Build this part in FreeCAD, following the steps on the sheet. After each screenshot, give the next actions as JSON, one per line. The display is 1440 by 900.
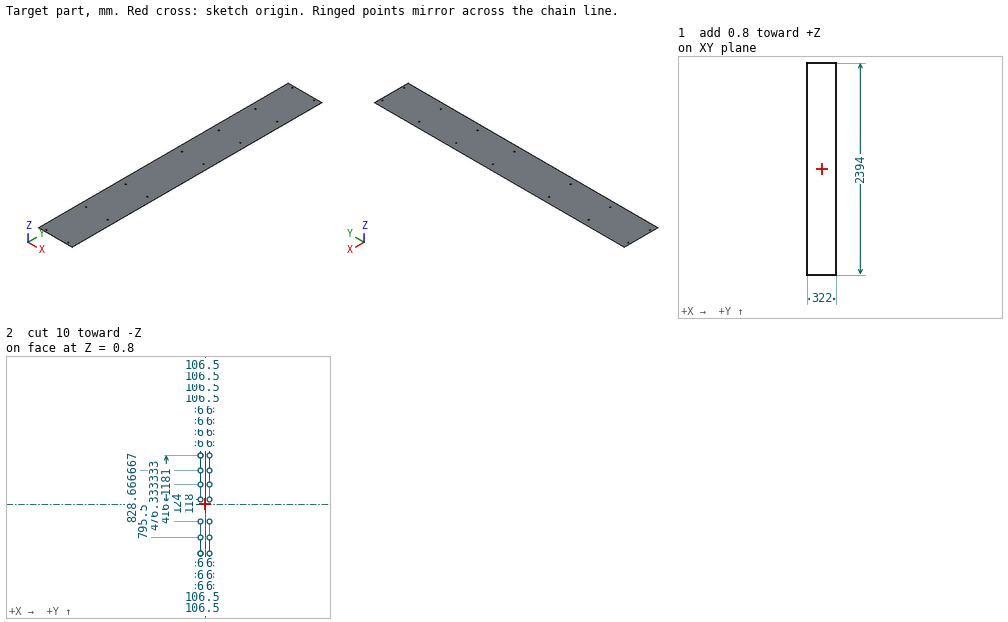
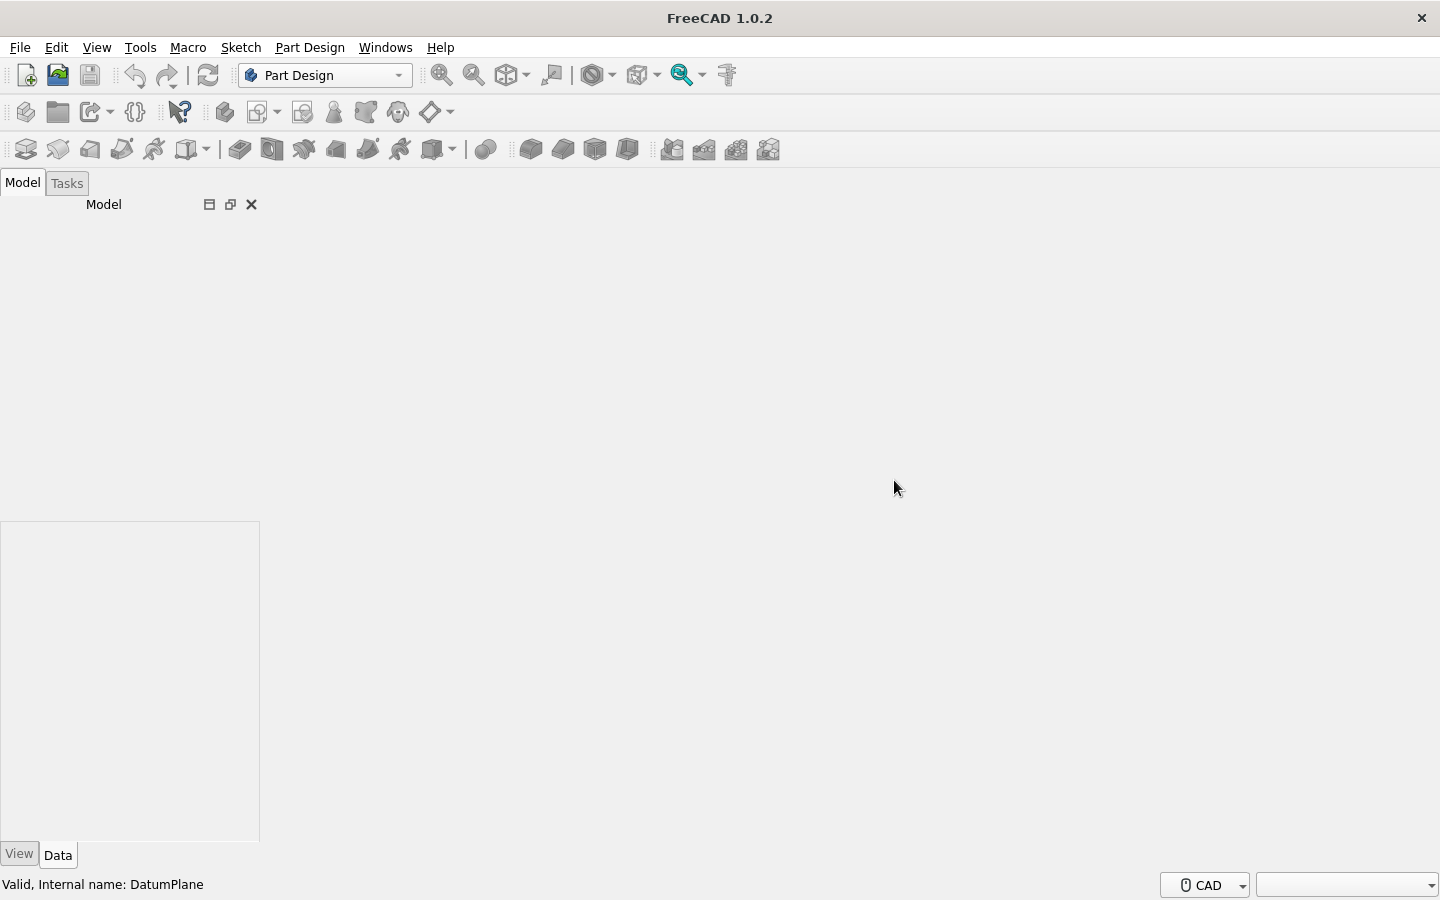
{"action": "left_click", "coordinate": [26, 76]}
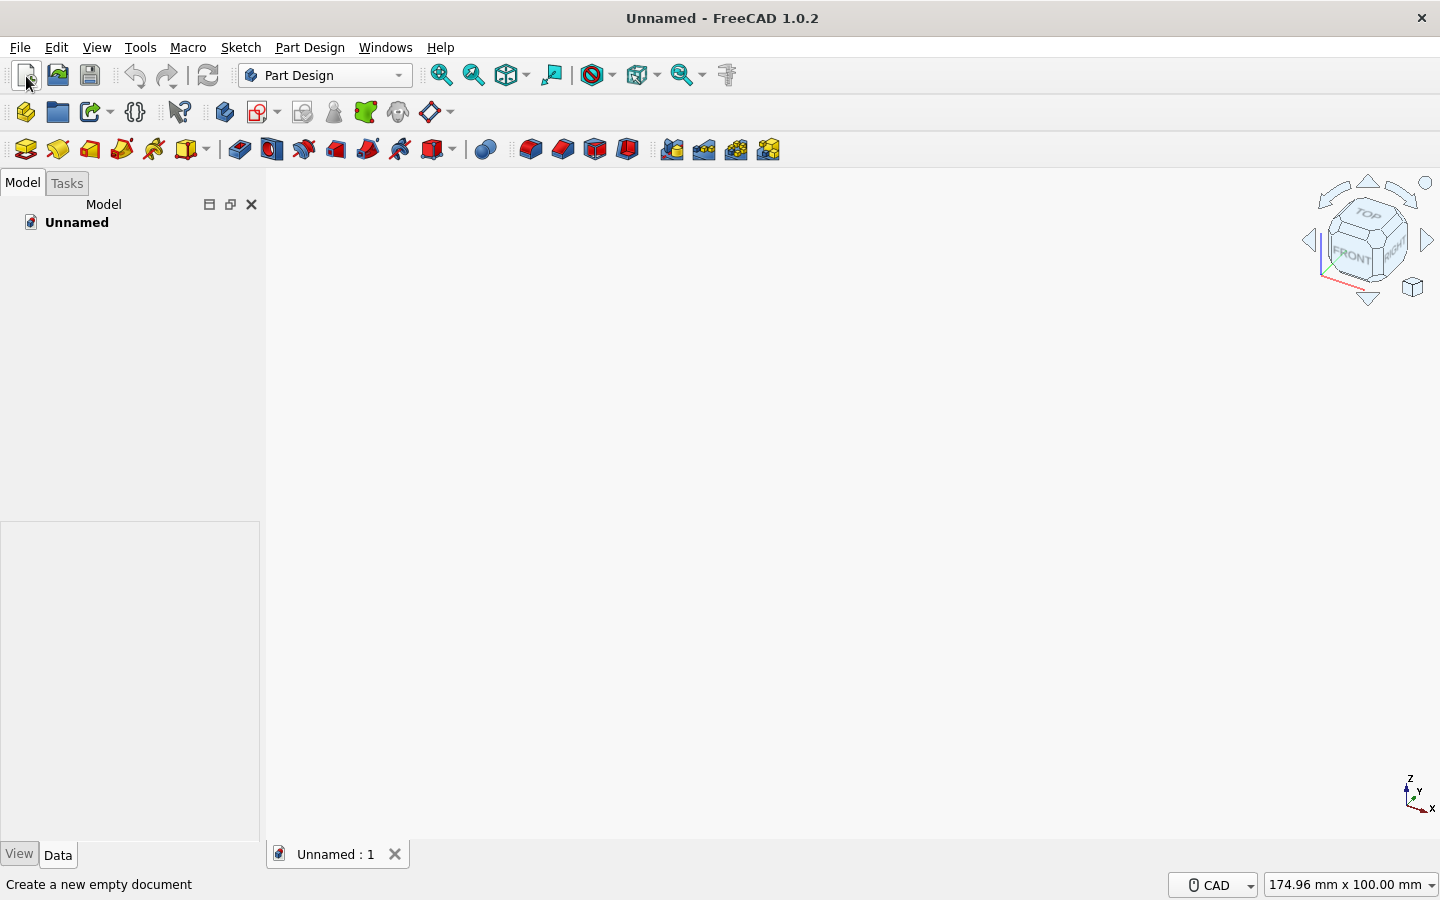
{"action": "left_click", "coordinate": [258, 112]}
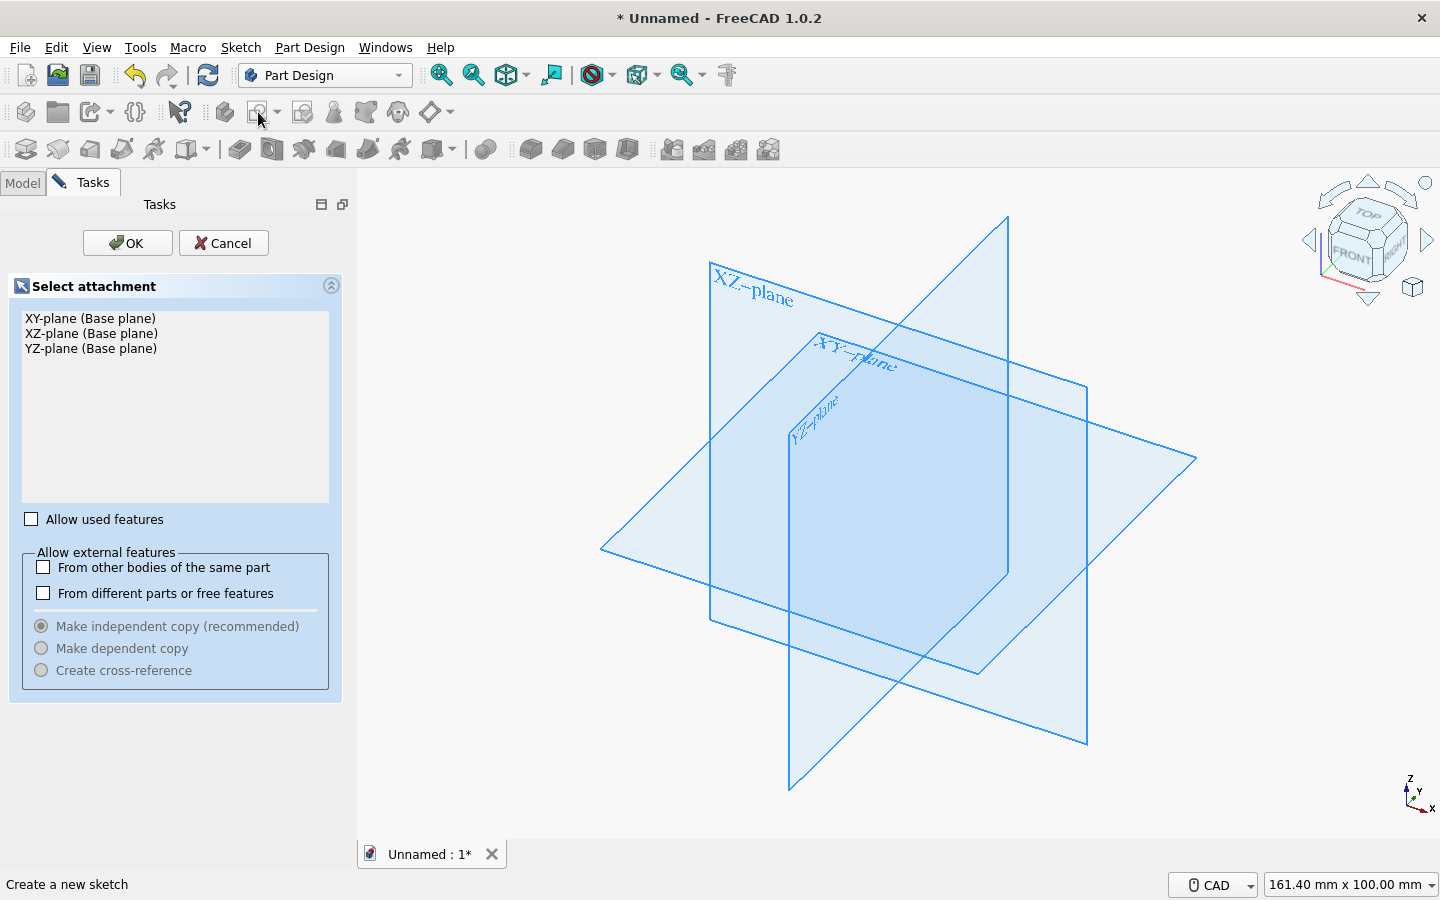
{"action": "left_click", "coordinate": [82, 318]}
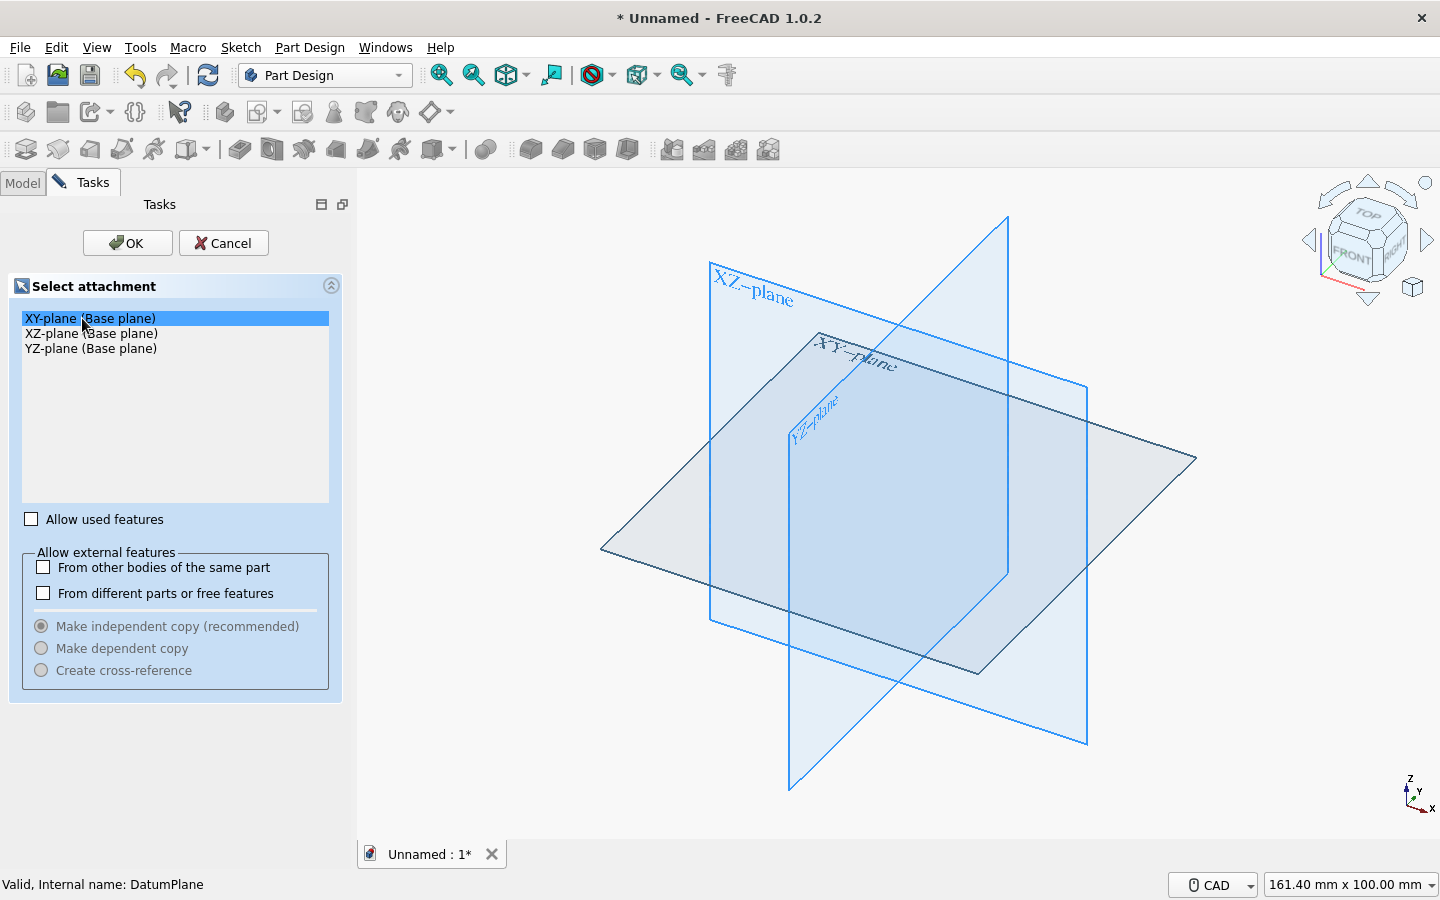
{"action": "left_click", "coordinate": [128, 243]}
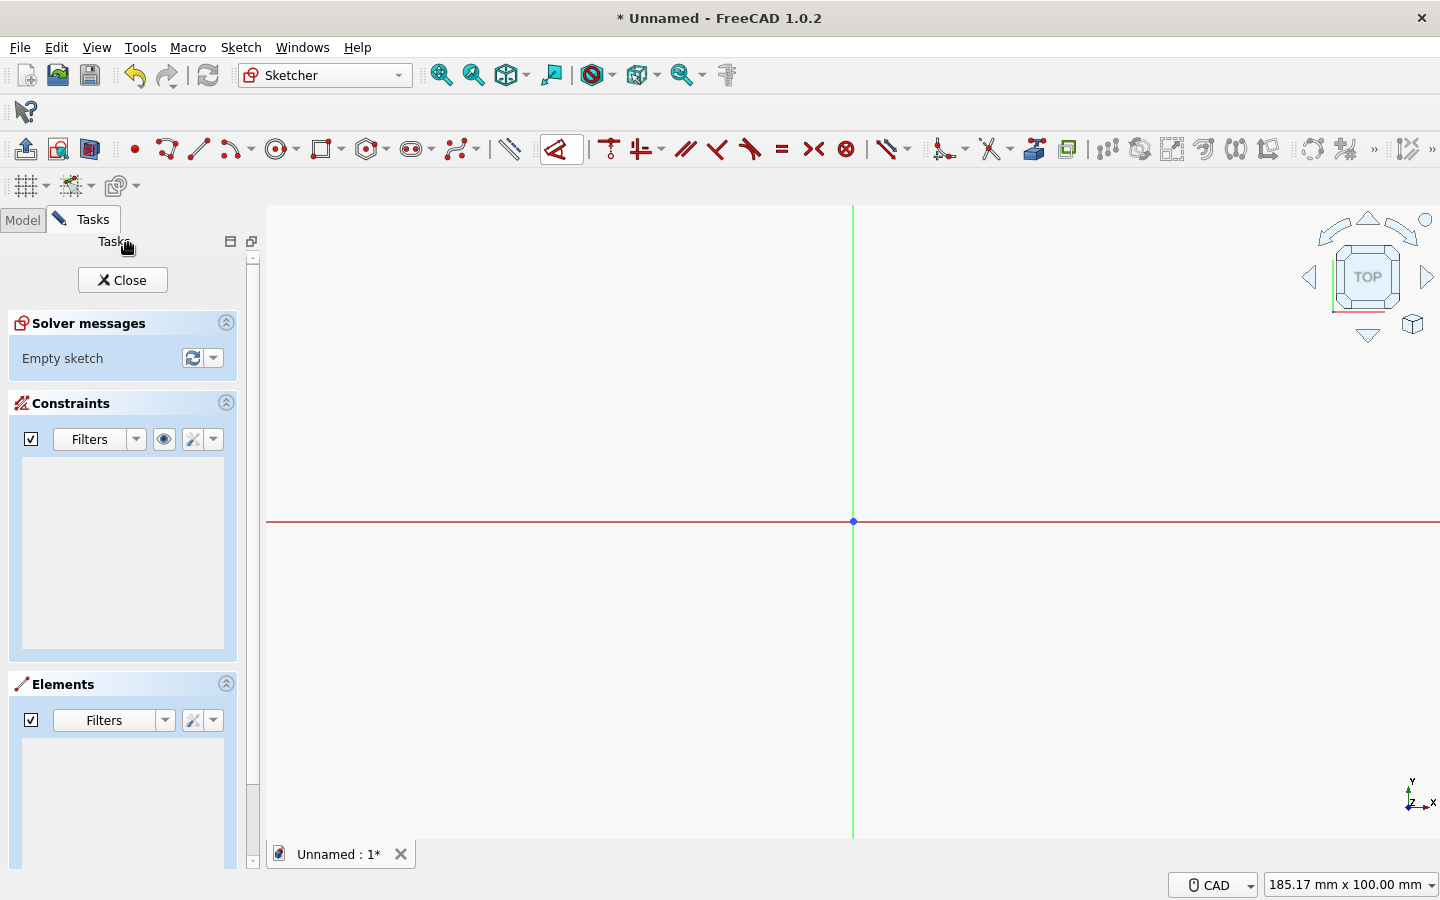
{"action": "scroll", "coordinate": [782, 522], "scroll_direction": "down", "scroll_amount": 17}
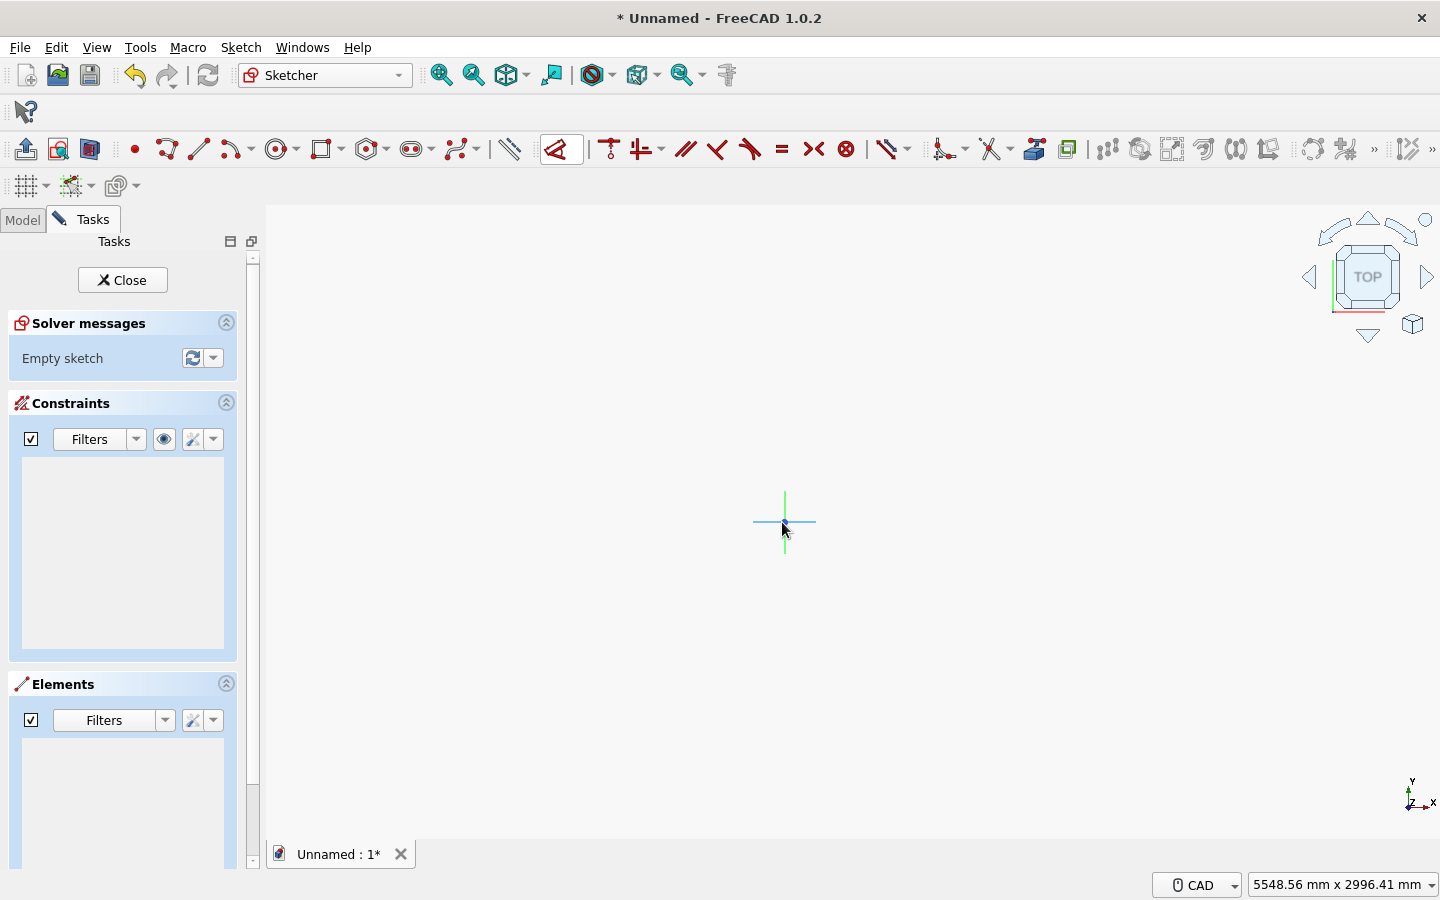
{"action": "key", "text": "g v"}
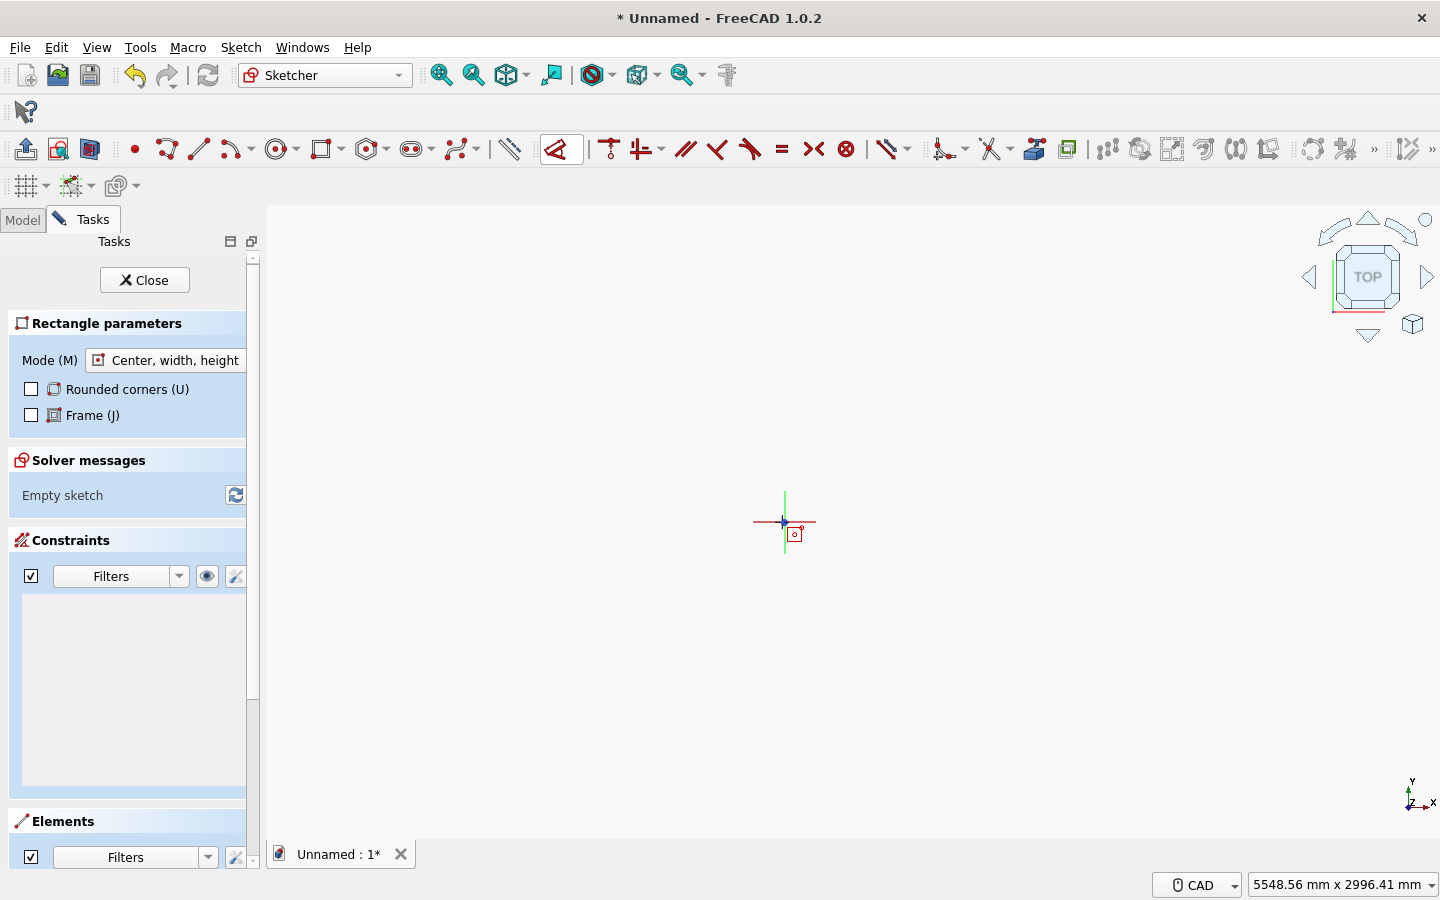
{"action": "left_click", "coordinate": [785, 522]}
{"action": "left_click", "coordinate": [819, 269]}
{"action": "key", "text": "Escape"}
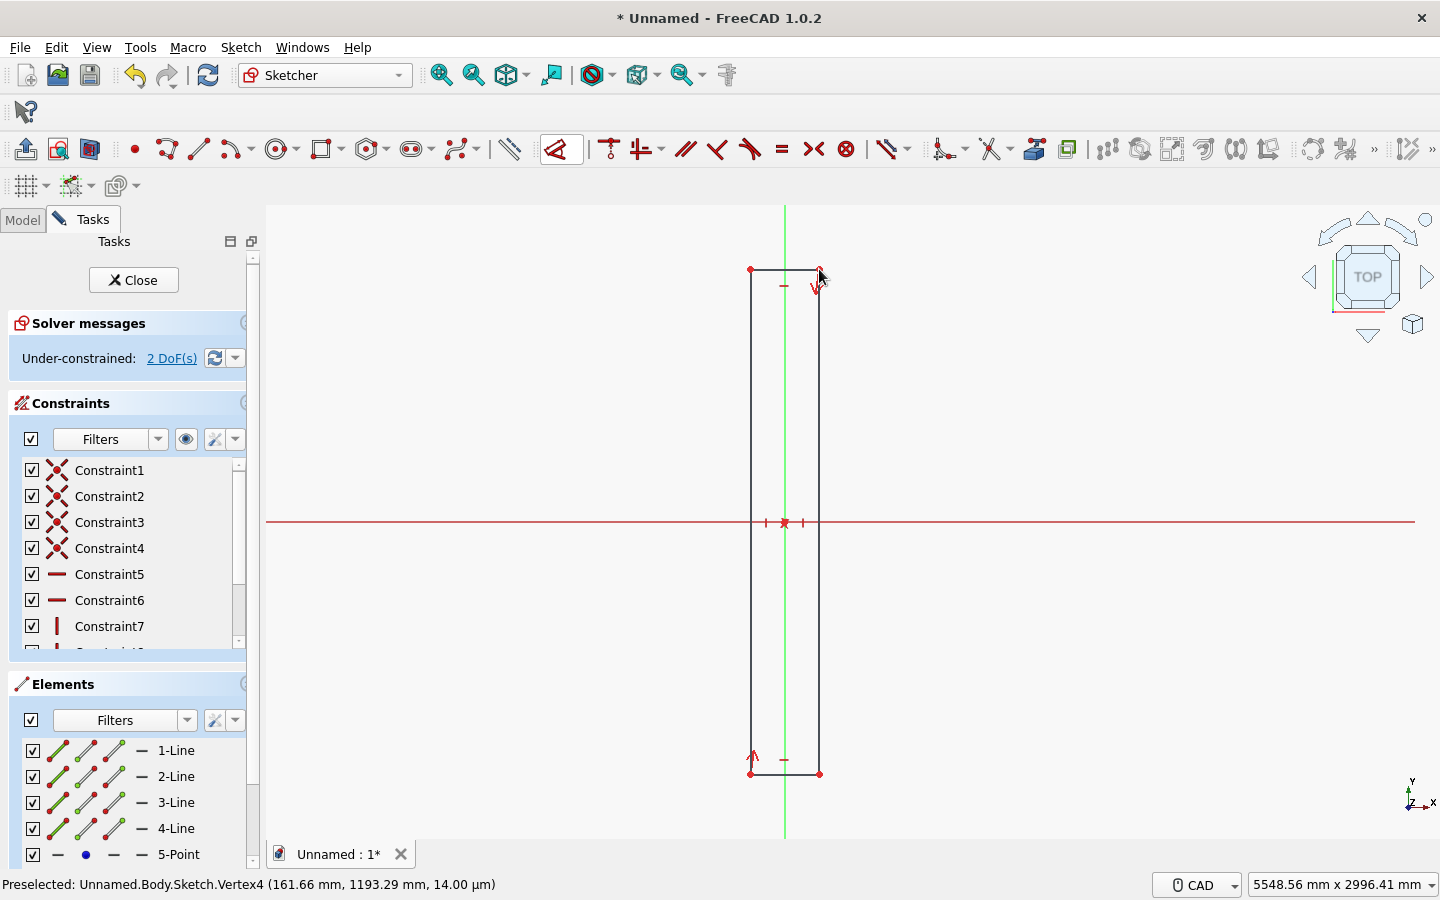
{"action": "left_click", "coordinate": [771, 775]}